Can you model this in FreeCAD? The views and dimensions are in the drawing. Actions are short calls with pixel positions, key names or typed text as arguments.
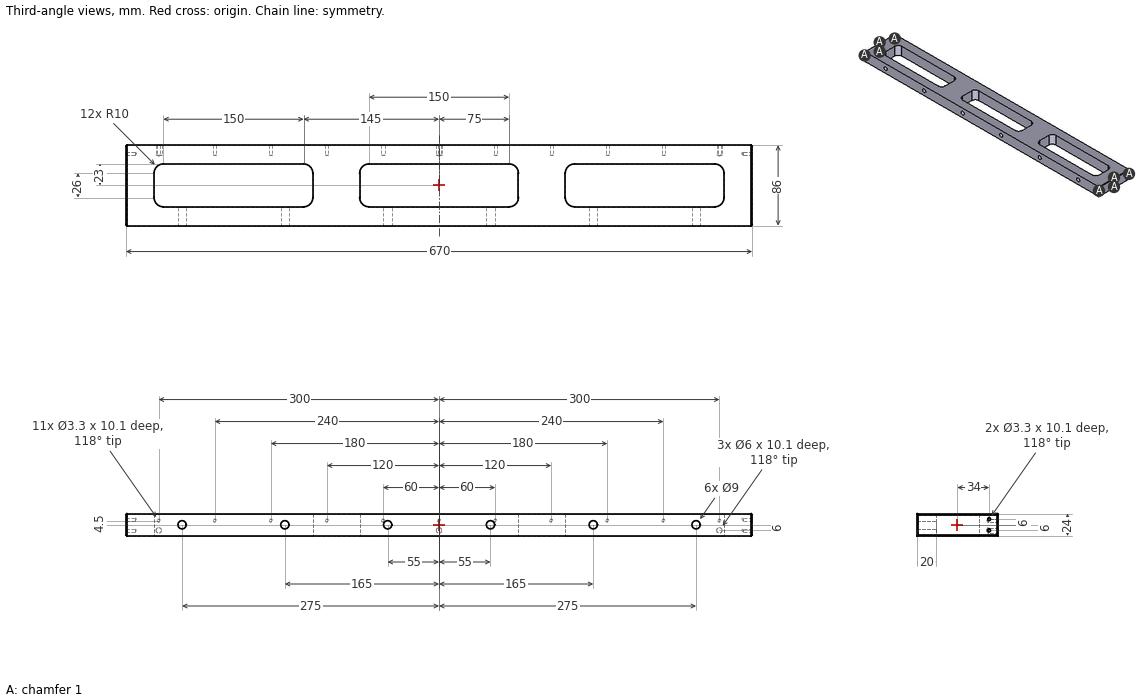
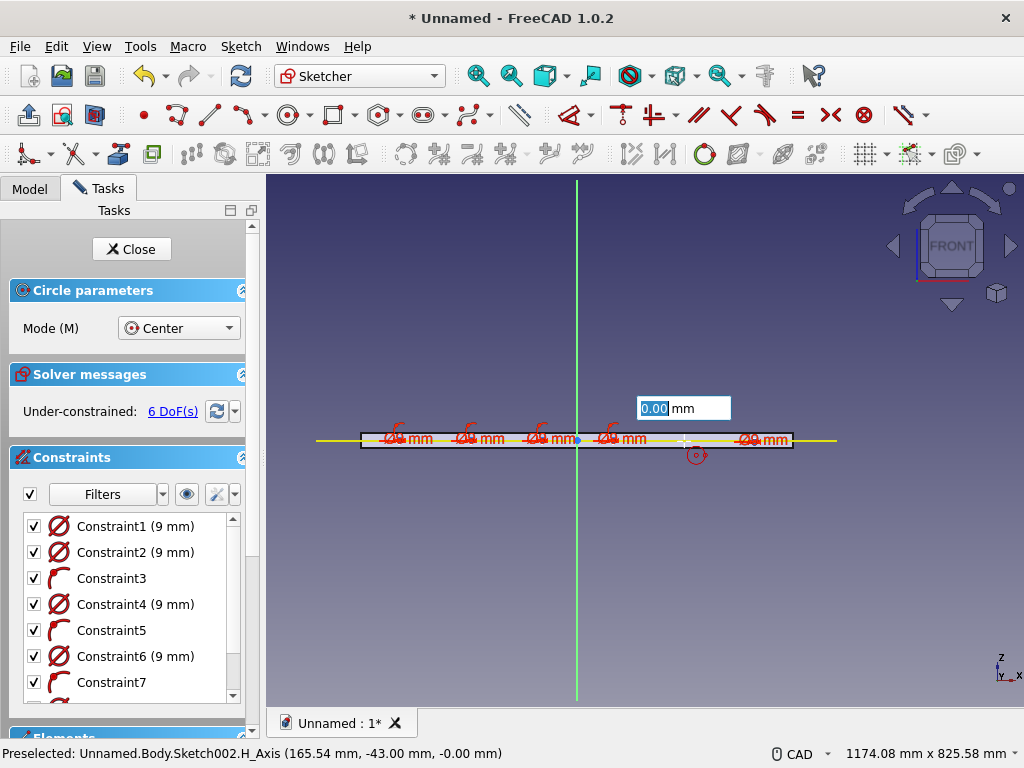
scroll(683, 443, up, 9)
move(678, 443)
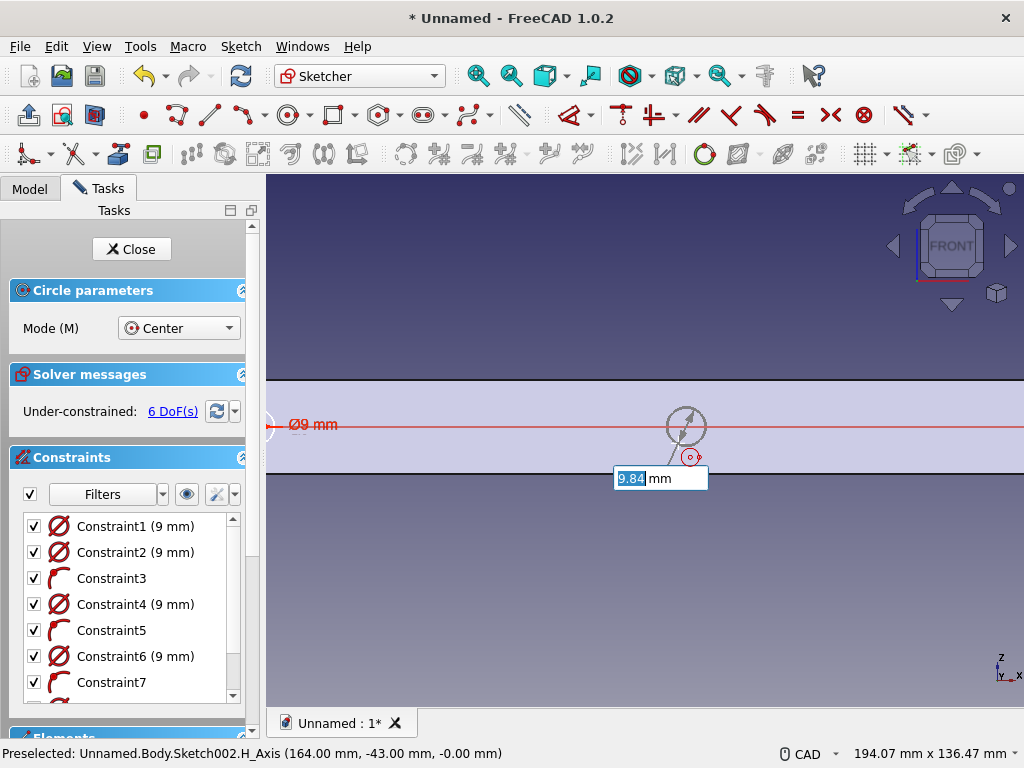
text(9)
key(Return)
key(Escape)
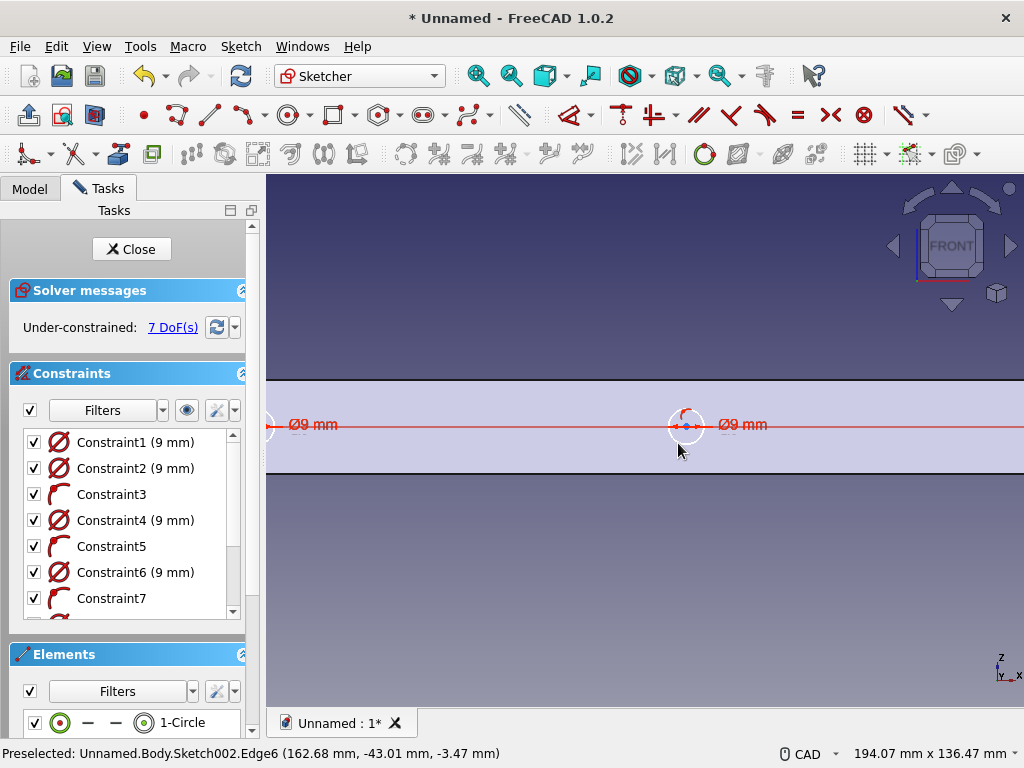
scroll(683, 443, down, 9)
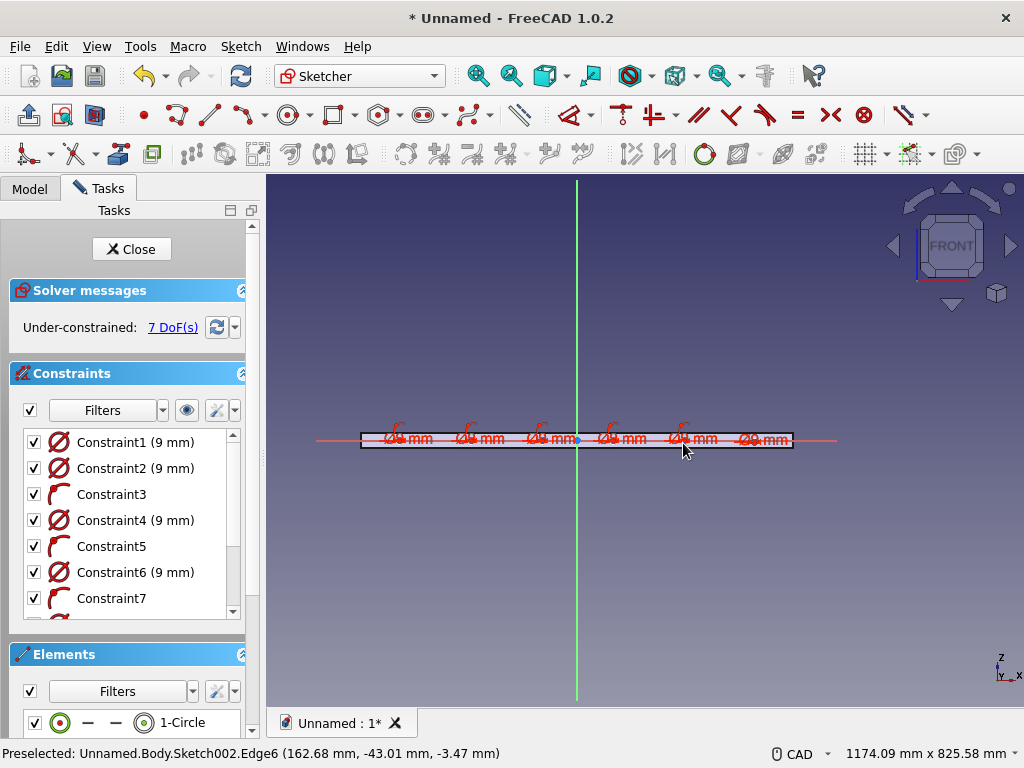
click(754, 442)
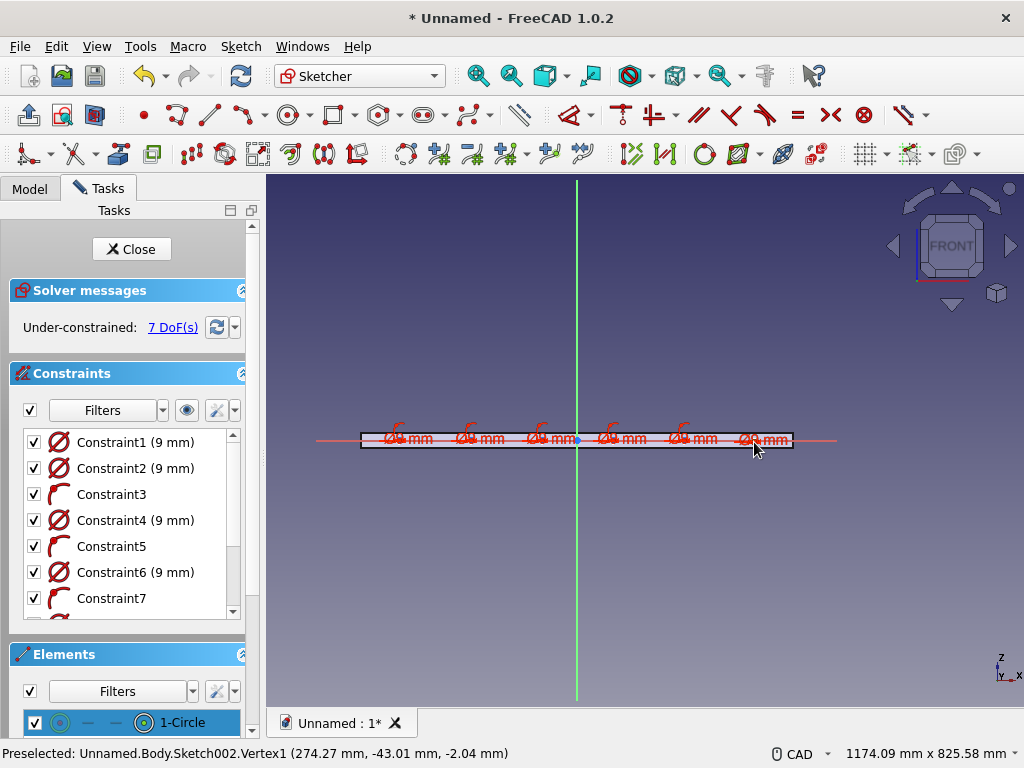
click(334, 441)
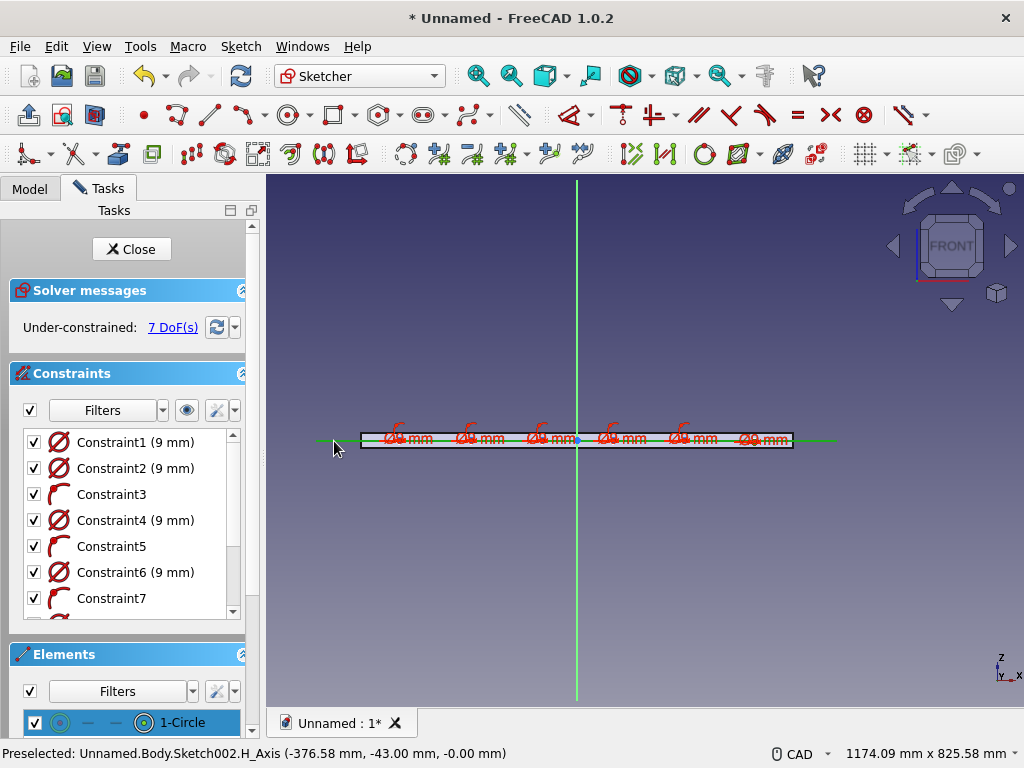
key(c)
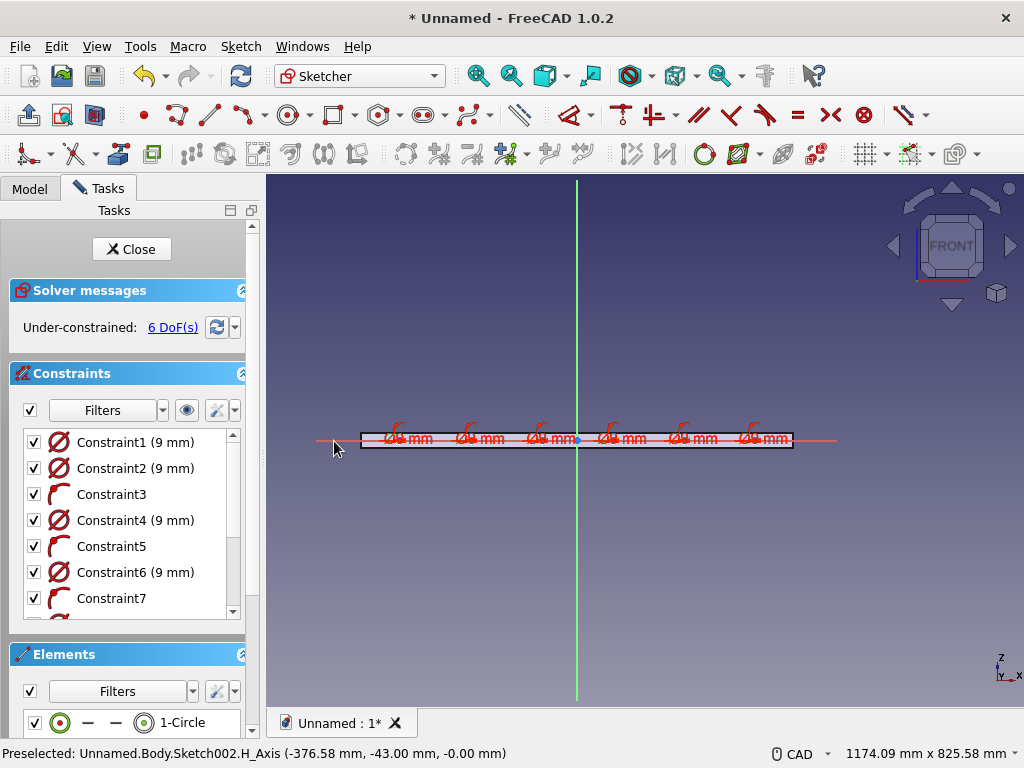
key(d)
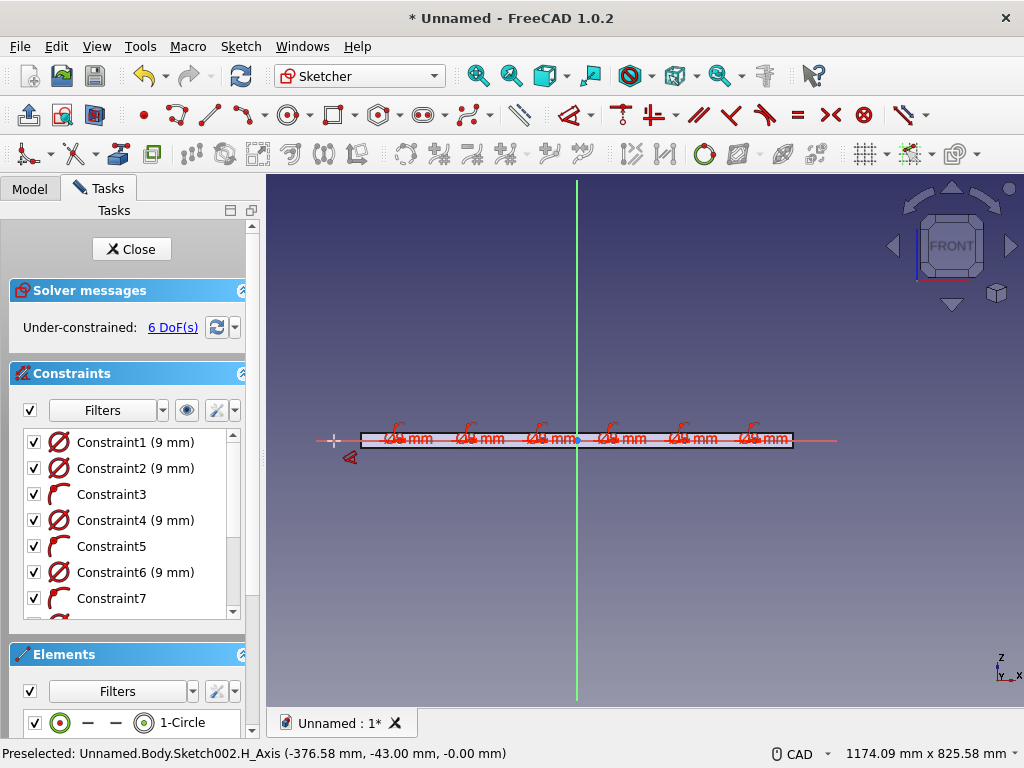
click(542, 441)
click(560, 475)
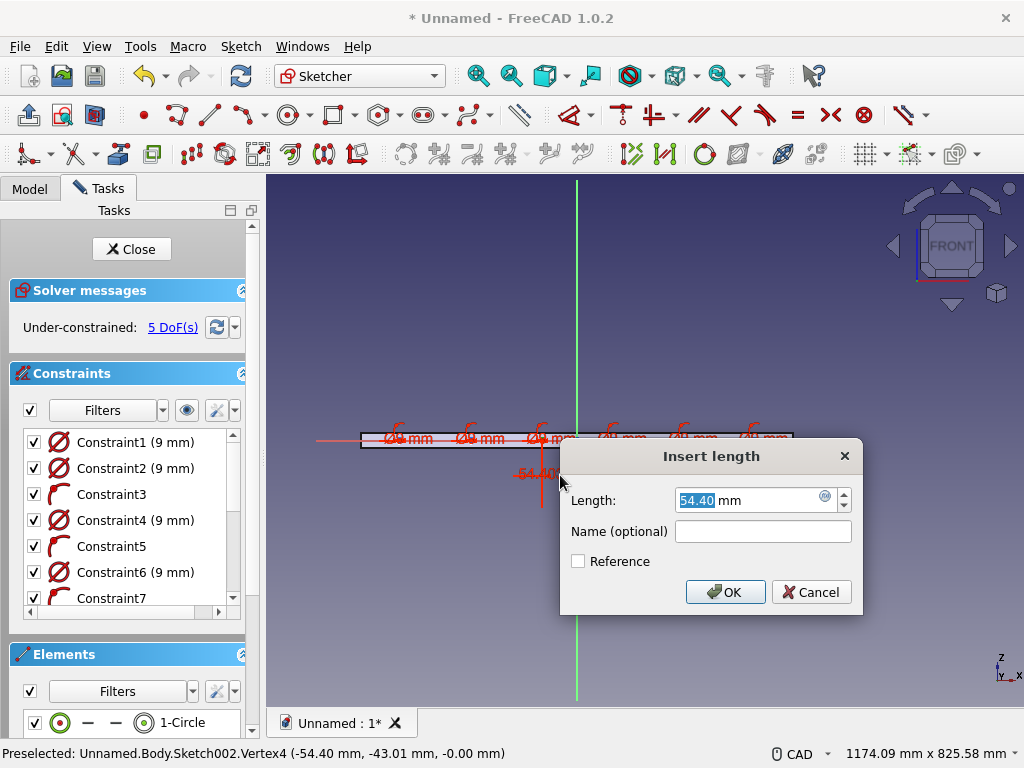
text(55)
key(Return)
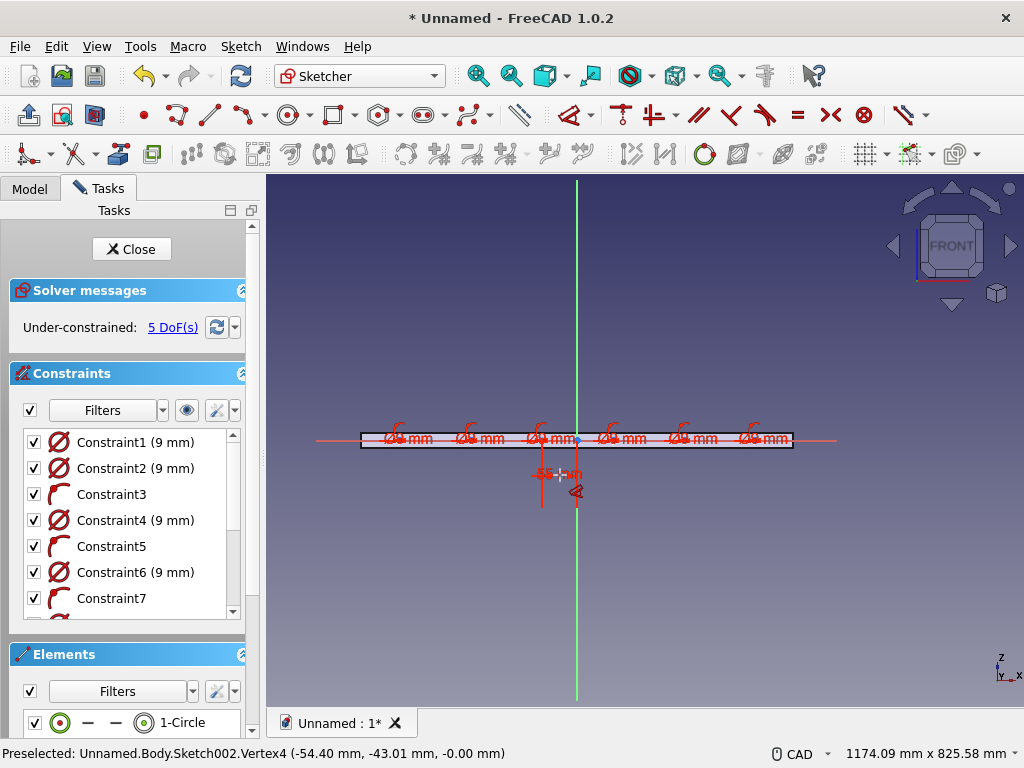
click(613, 441)
click(595, 407)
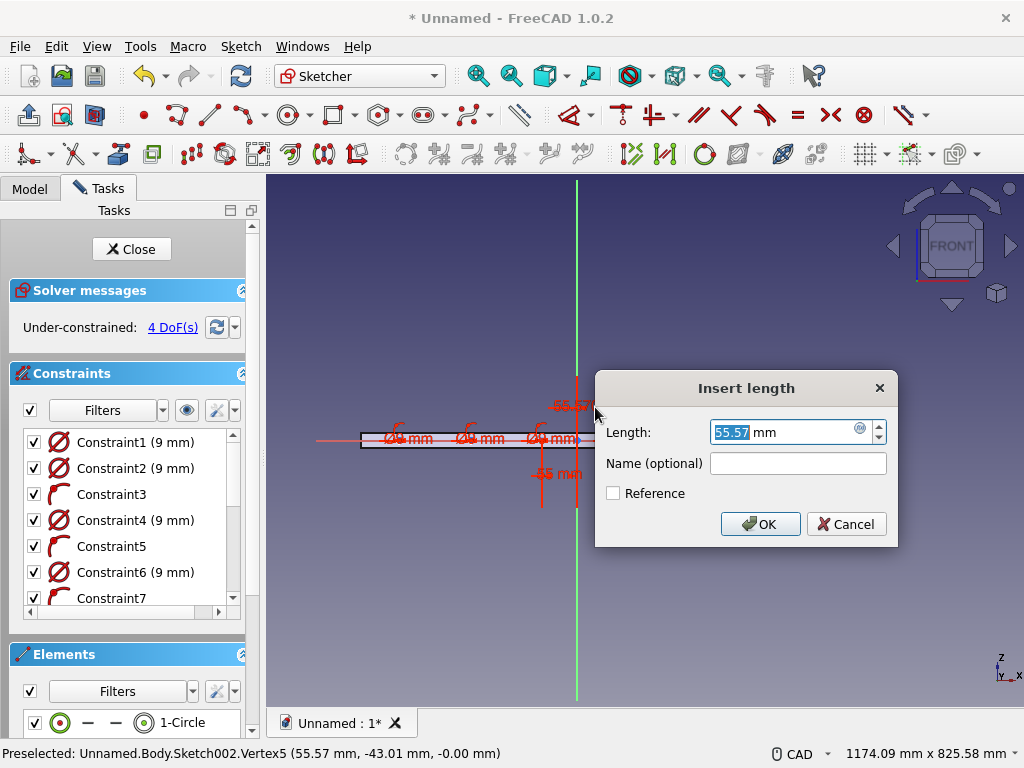
text(55)
key(Return)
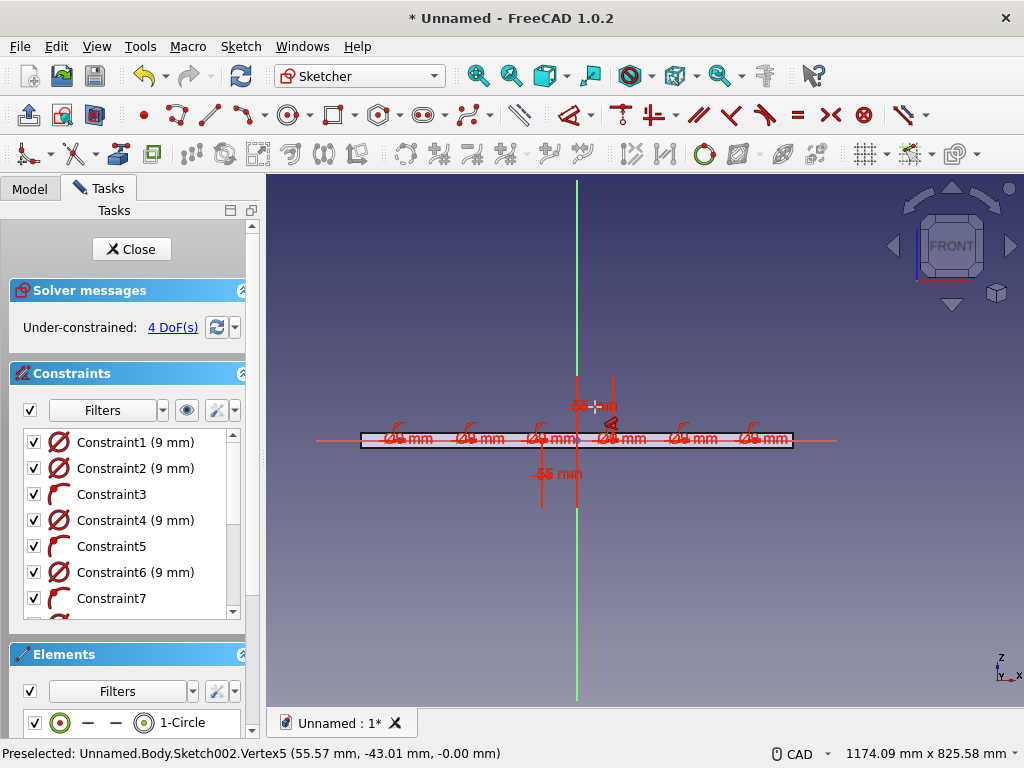
click(754, 441)
click(666, 475)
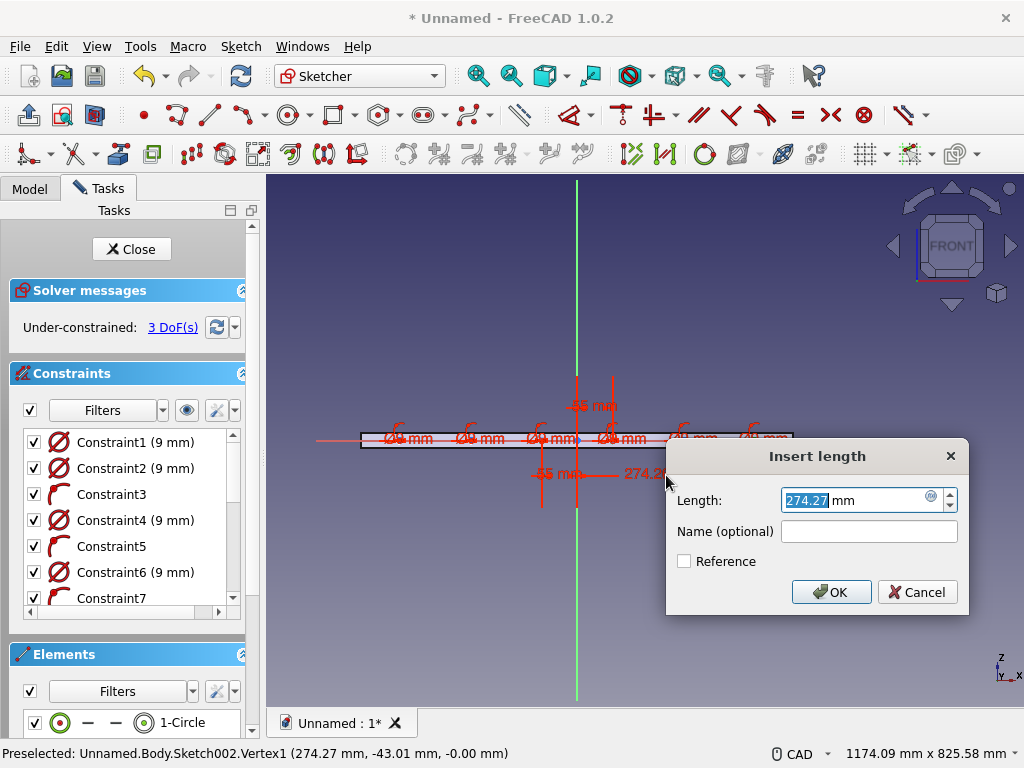
text(275)
key(Return)